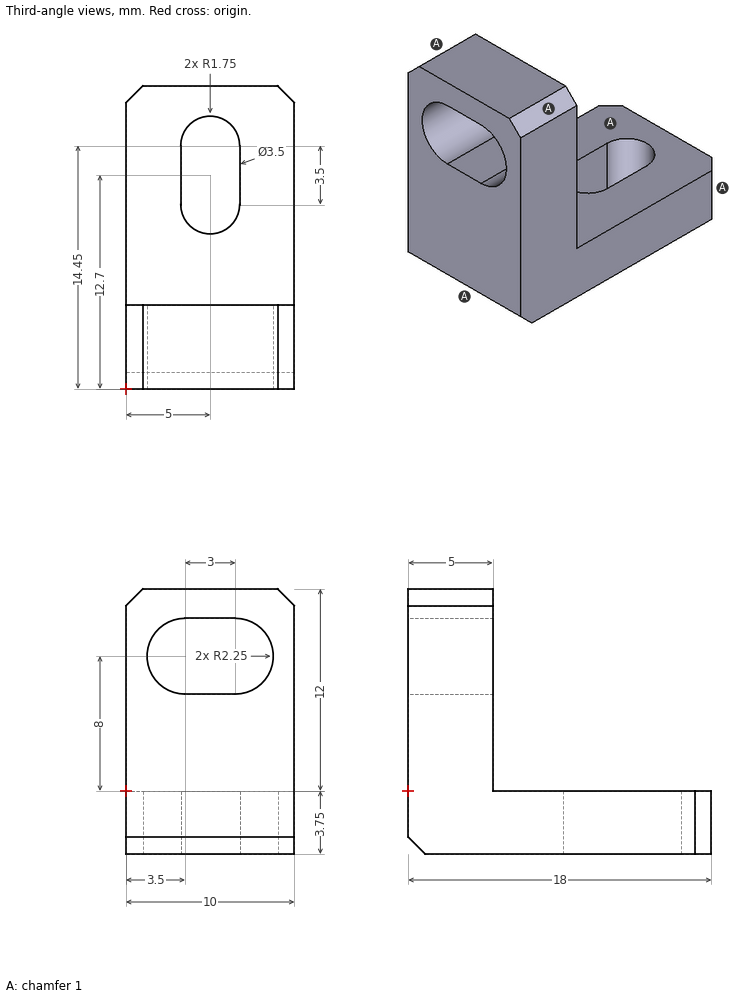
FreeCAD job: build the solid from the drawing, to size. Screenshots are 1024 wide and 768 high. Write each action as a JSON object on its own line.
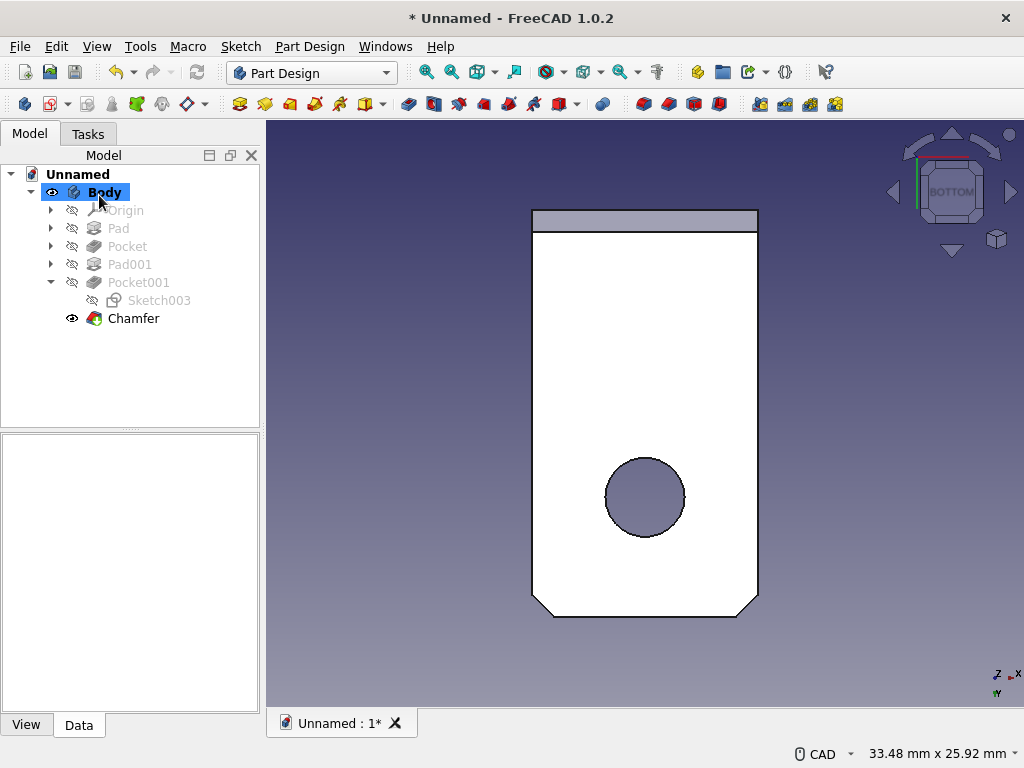
{"action": "key", "text": "0"}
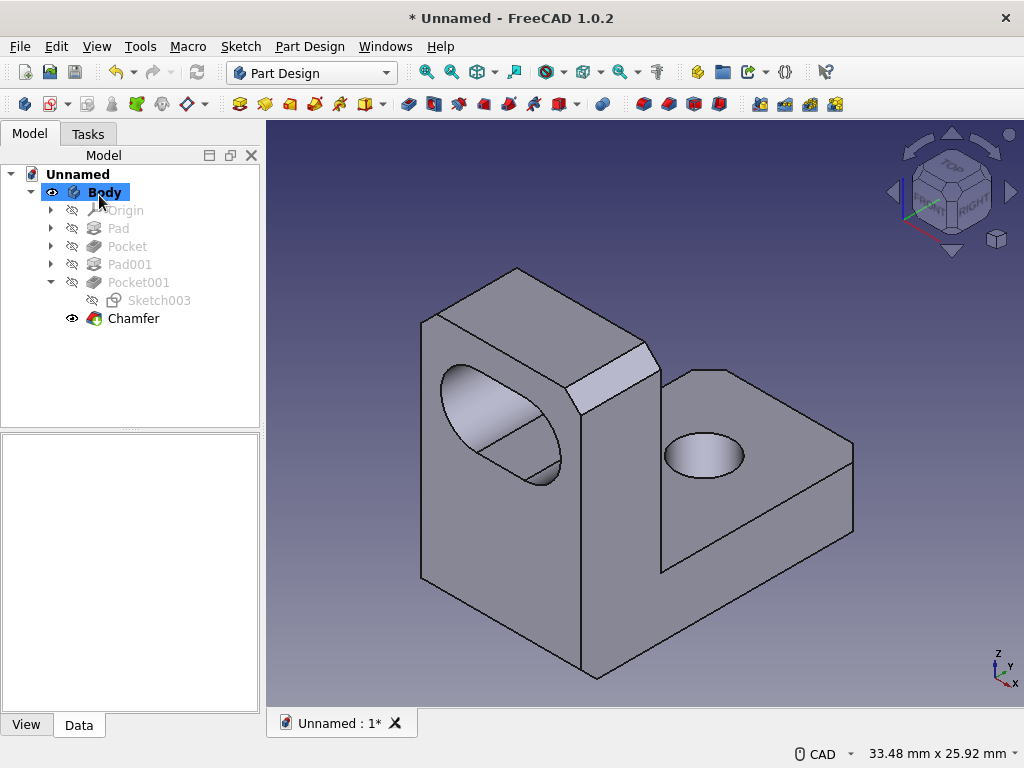
{"action": "left_click", "coordinate": [701, 509]}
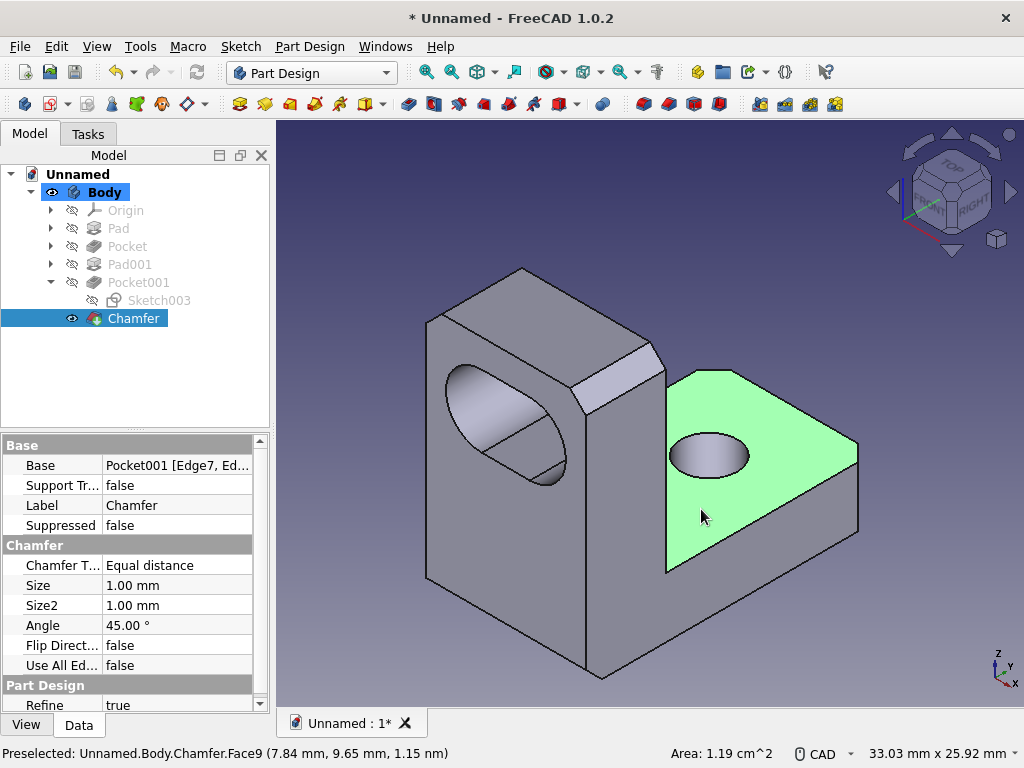
{"action": "left_click", "coordinate": [50, 104]}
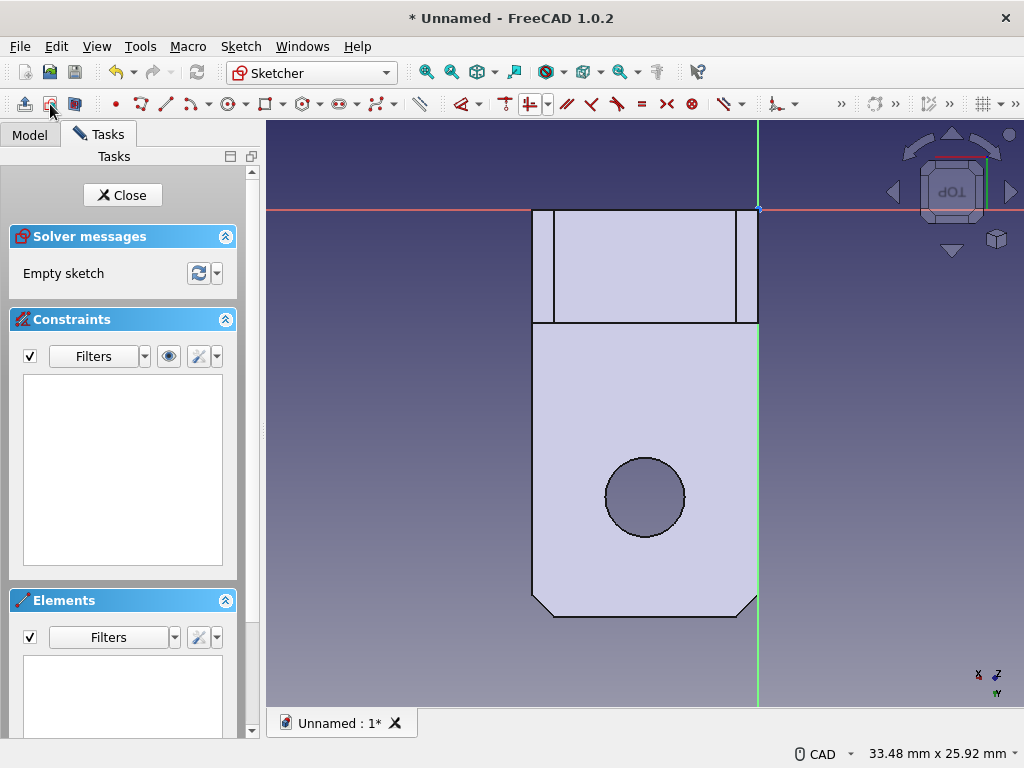
{"action": "left_click", "coordinate": [75, 104]}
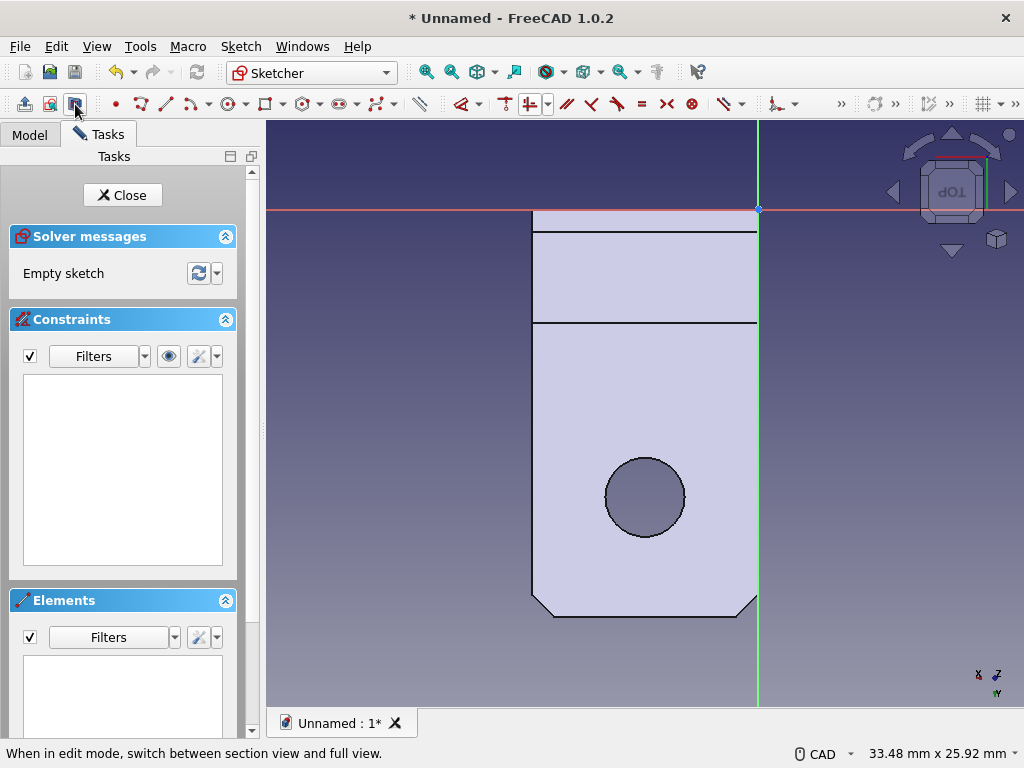
{"action": "key", "text": "g s"}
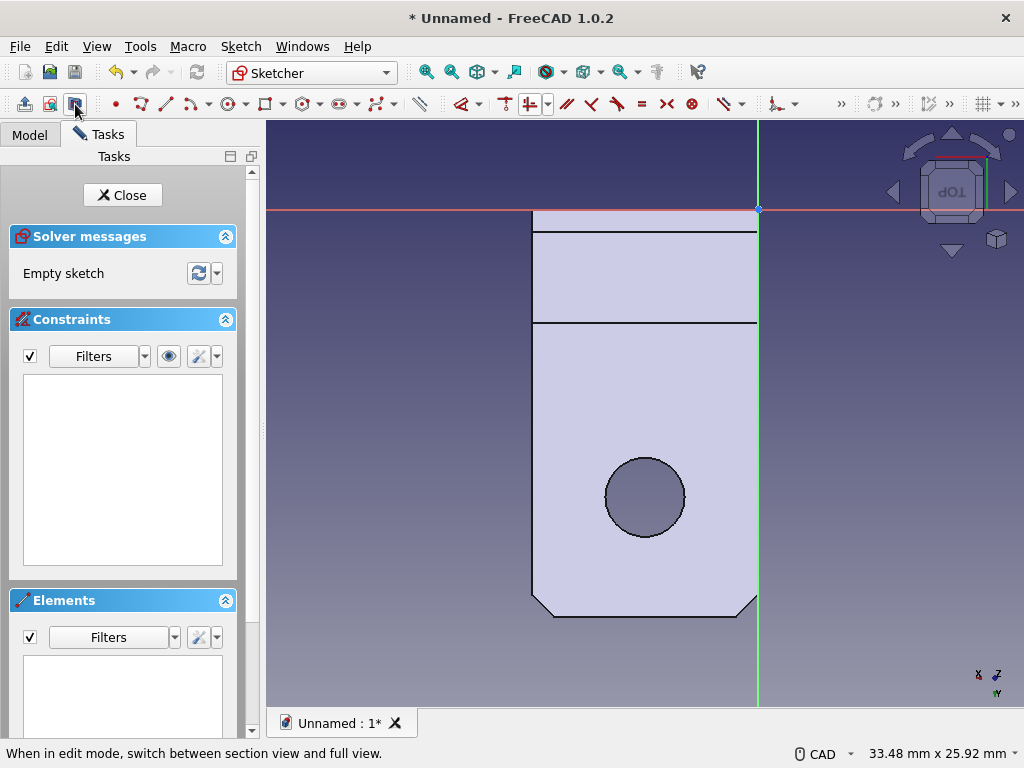
{"action": "left_click", "coordinate": [645, 537]}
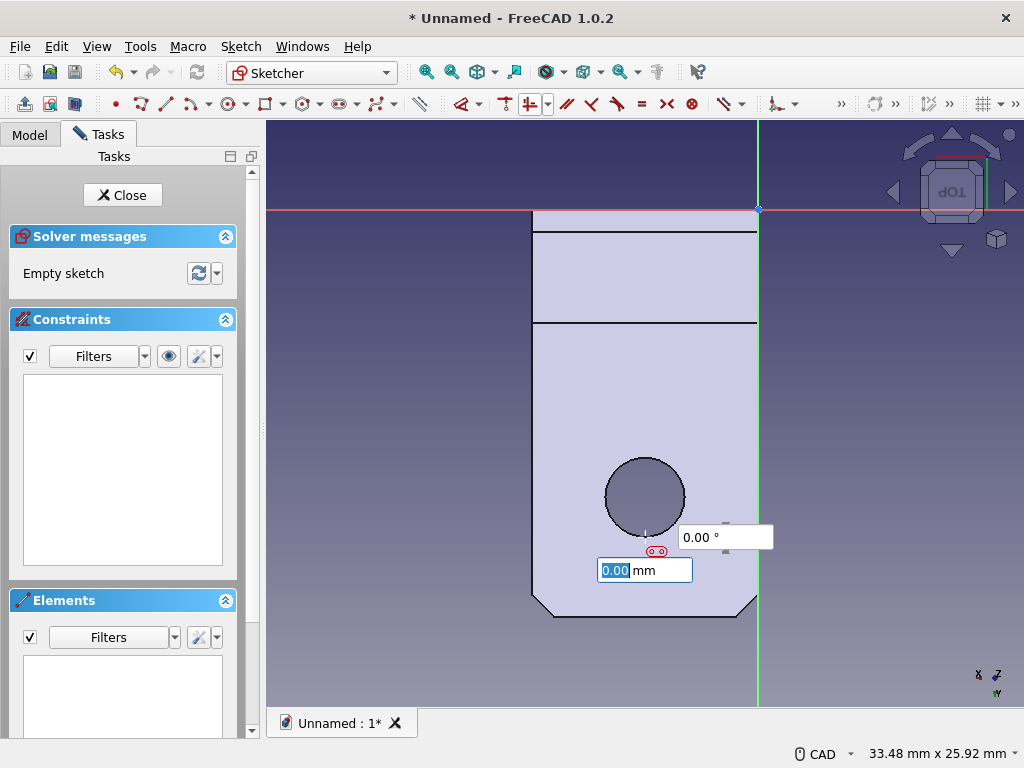
{"action": "left_click", "coordinate": [645, 458]}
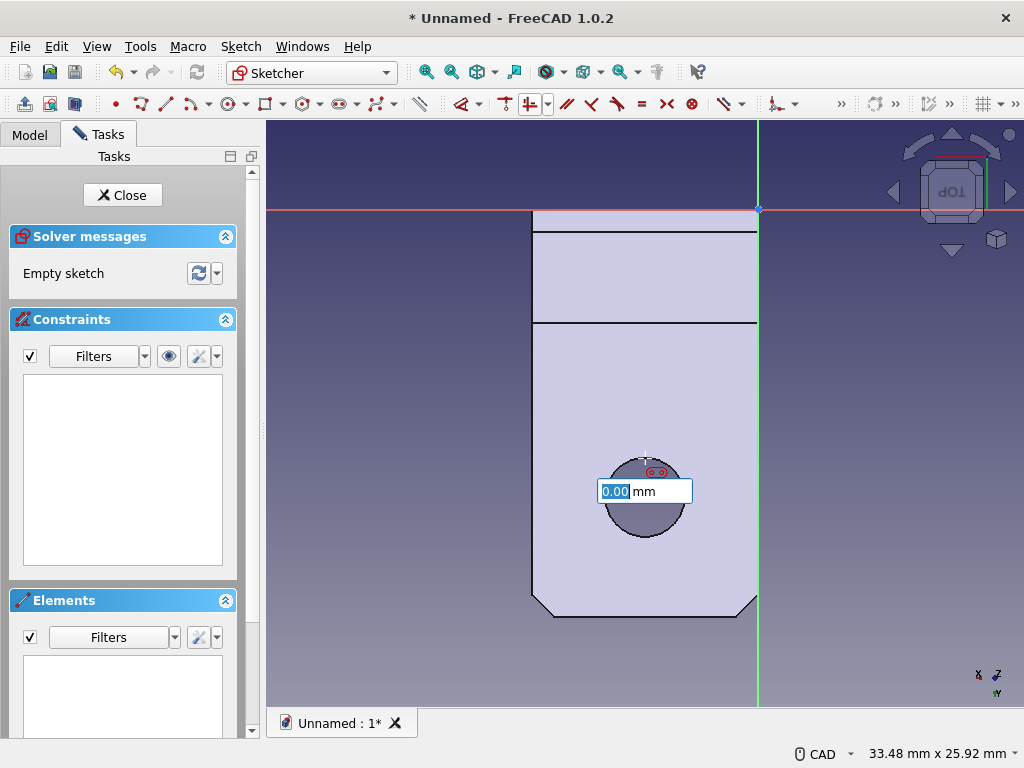
{"action": "left_click", "coordinate": [605, 497]}
{"action": "key", "text": "Escape"}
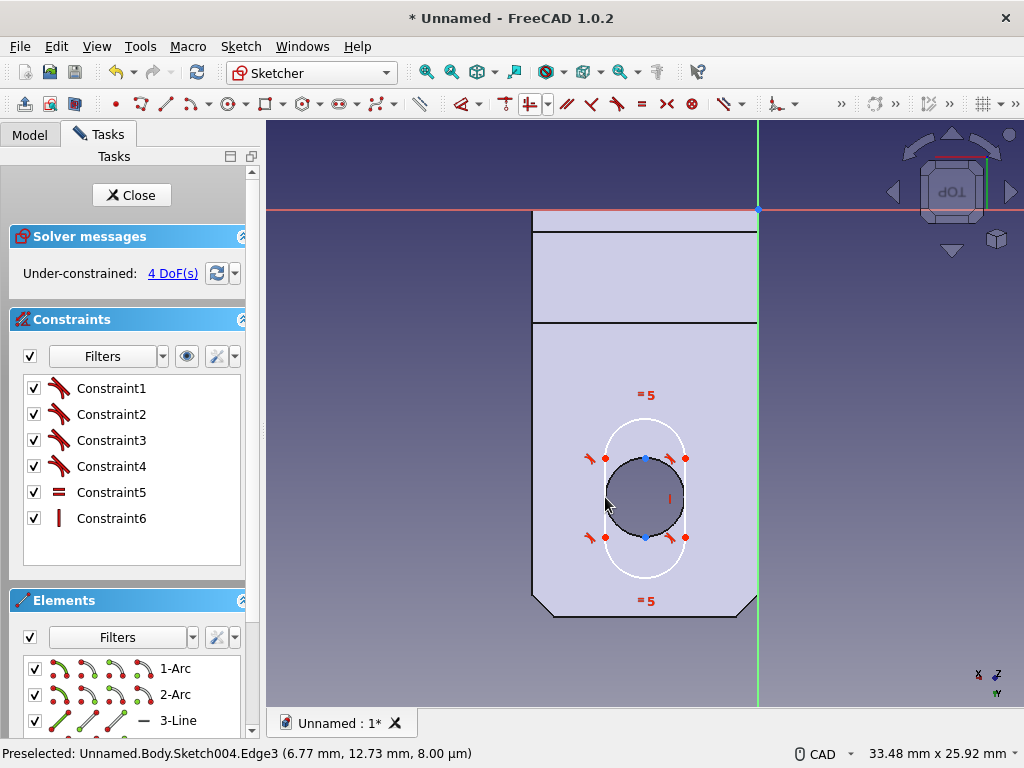
{"action": "left_click", "coordinate": [460, 104]}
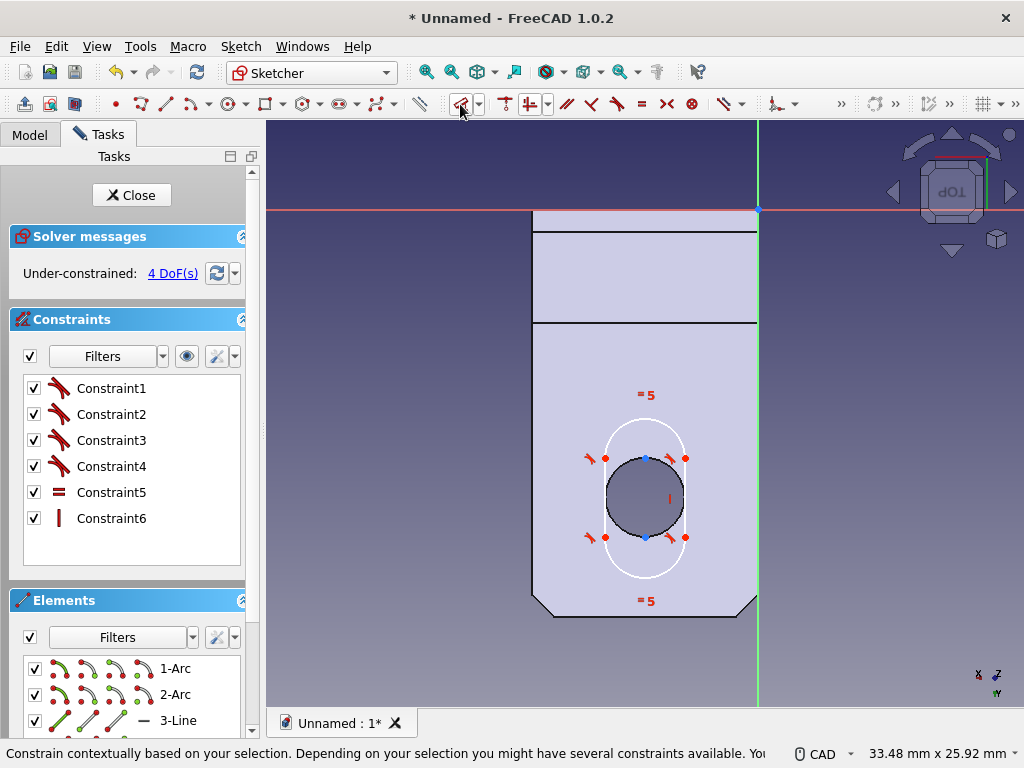
{"action": "left_click", "coordinate": [621, 570]}
{"action": "left_click", "coordinate": [602, 596]}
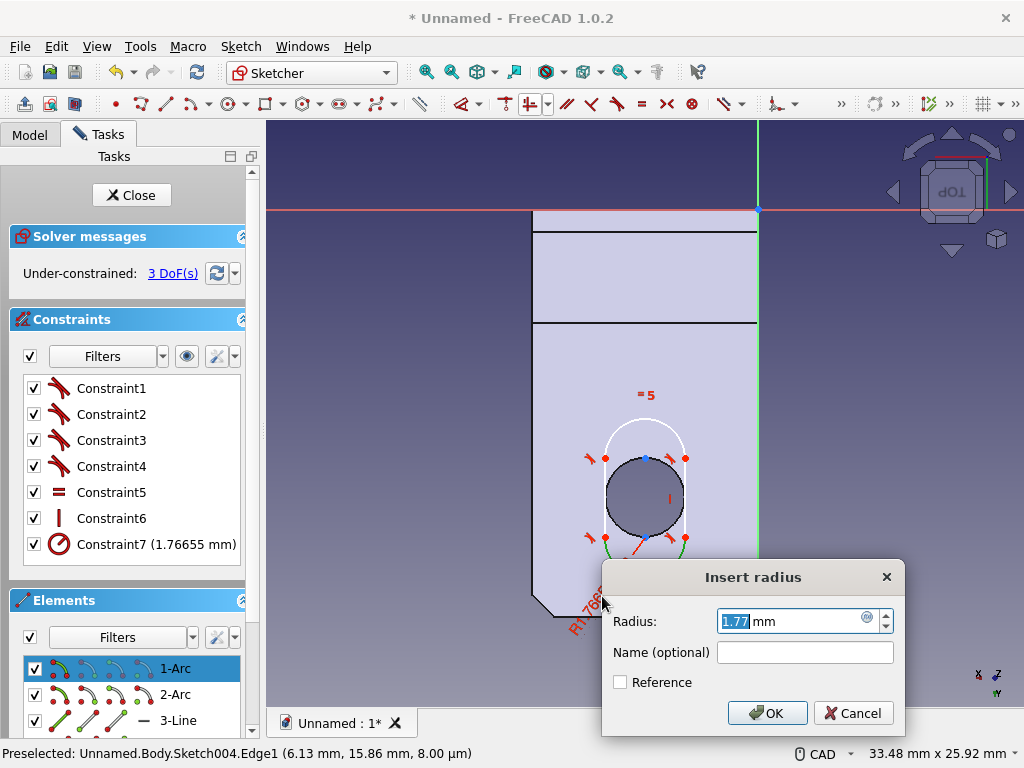
{"action": "type", "text": "1.75"}
{"action": "key", "text": "Return"}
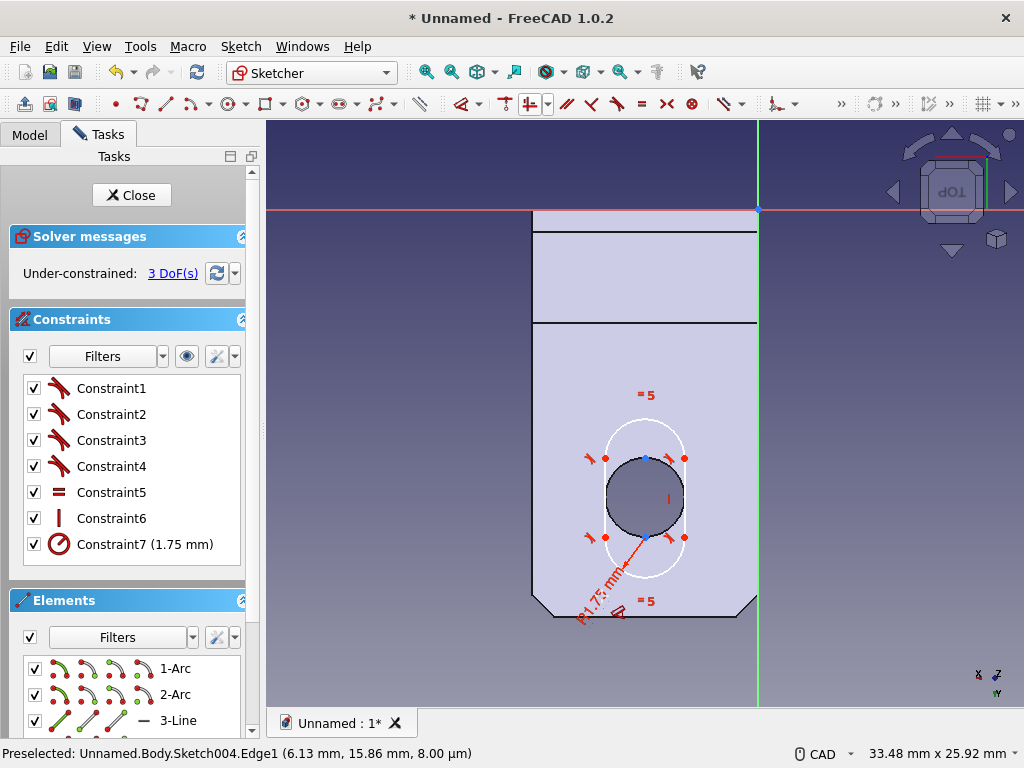
{"action": "left_click", "coordinate": [645, 538]}
{"action": "left_click", "coordinate": [702, 176]}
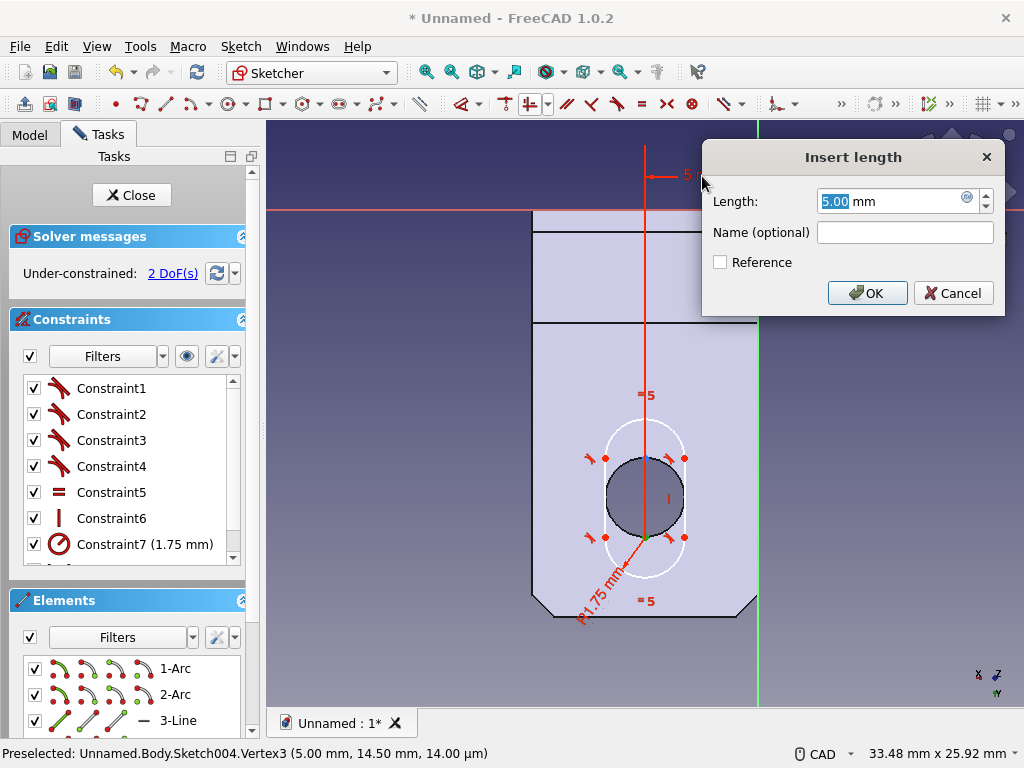
{"action": "type", "text": "5"}
{"action": "key", "text": "Return"}